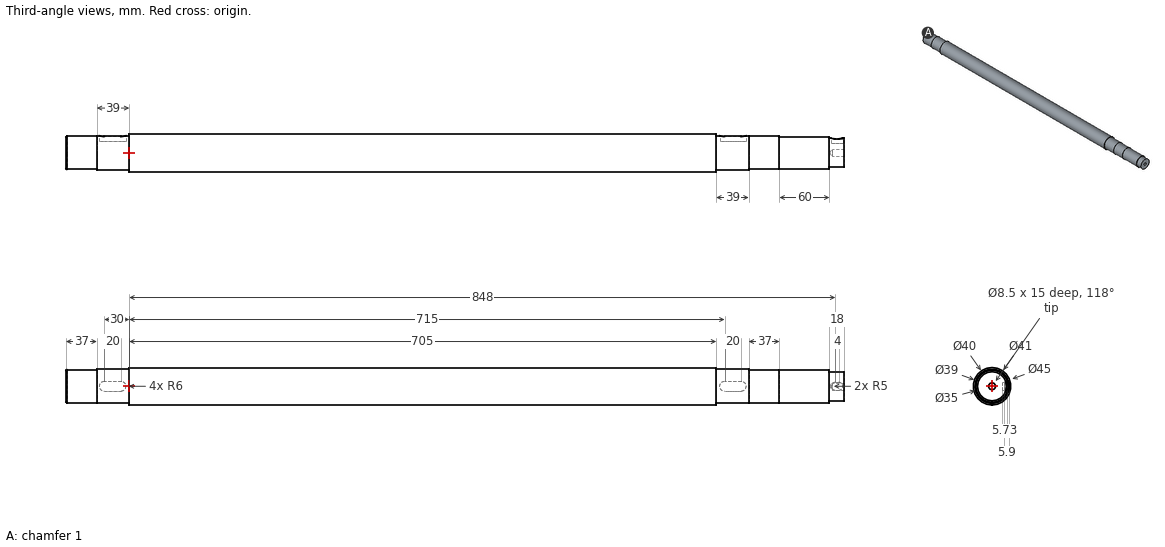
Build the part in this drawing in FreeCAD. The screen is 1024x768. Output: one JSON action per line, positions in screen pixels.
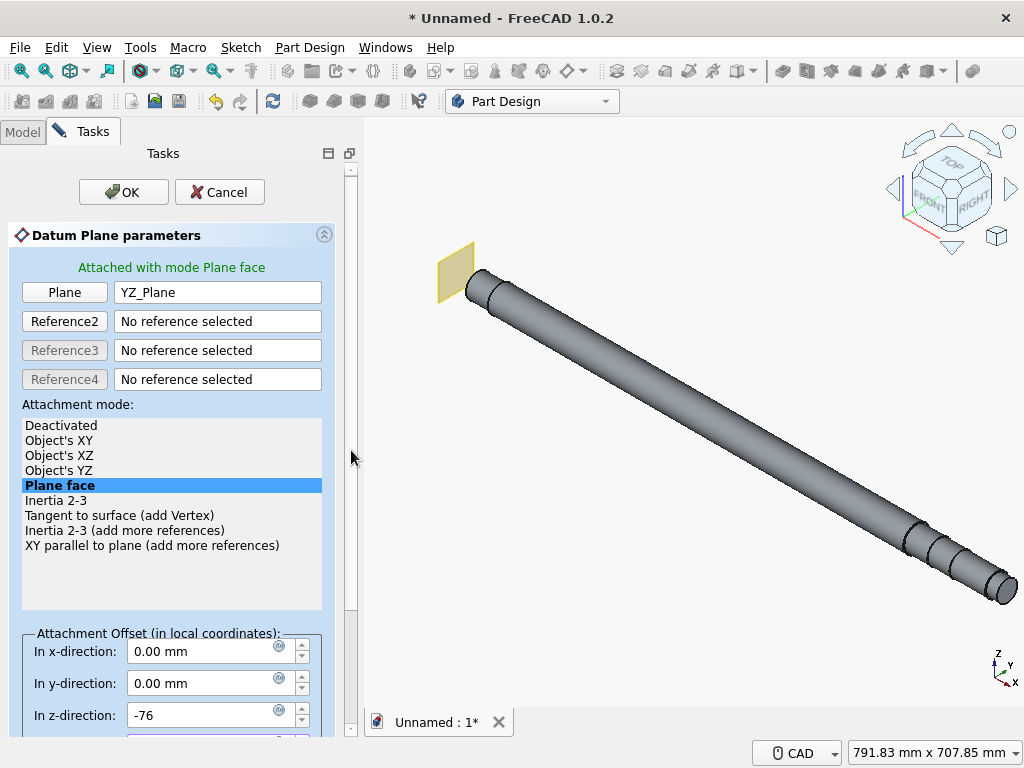
{"action": "left_click", "coordinate": [124, 192]}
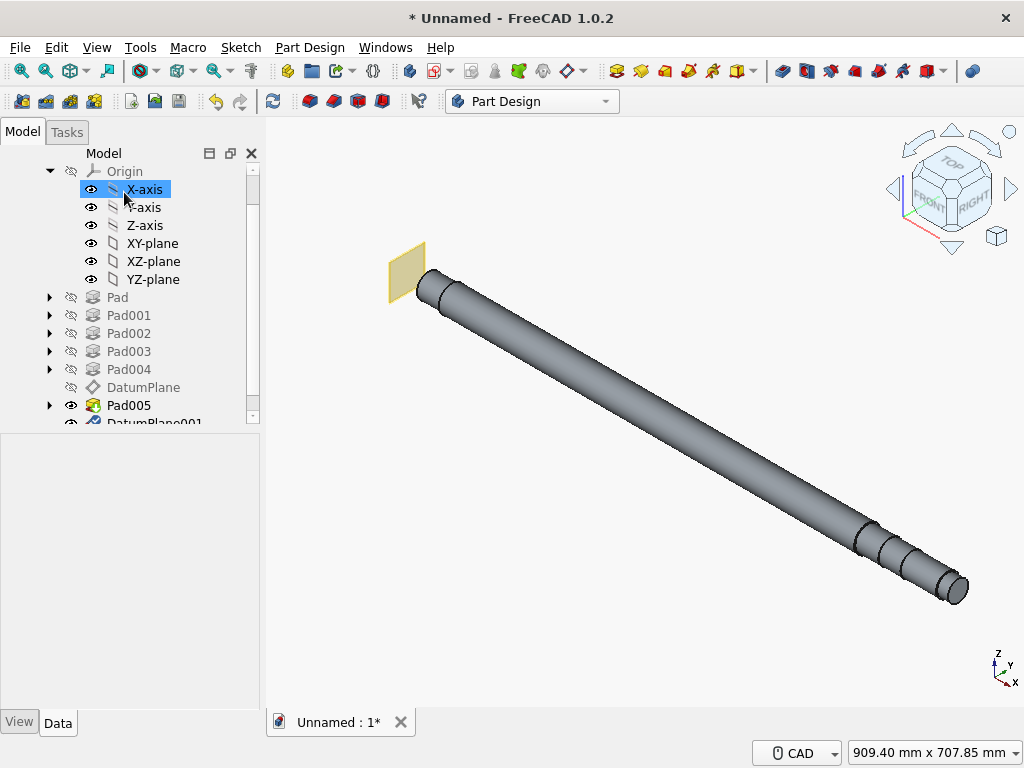
{"action": "left_click", "coordinate": [116, 423]}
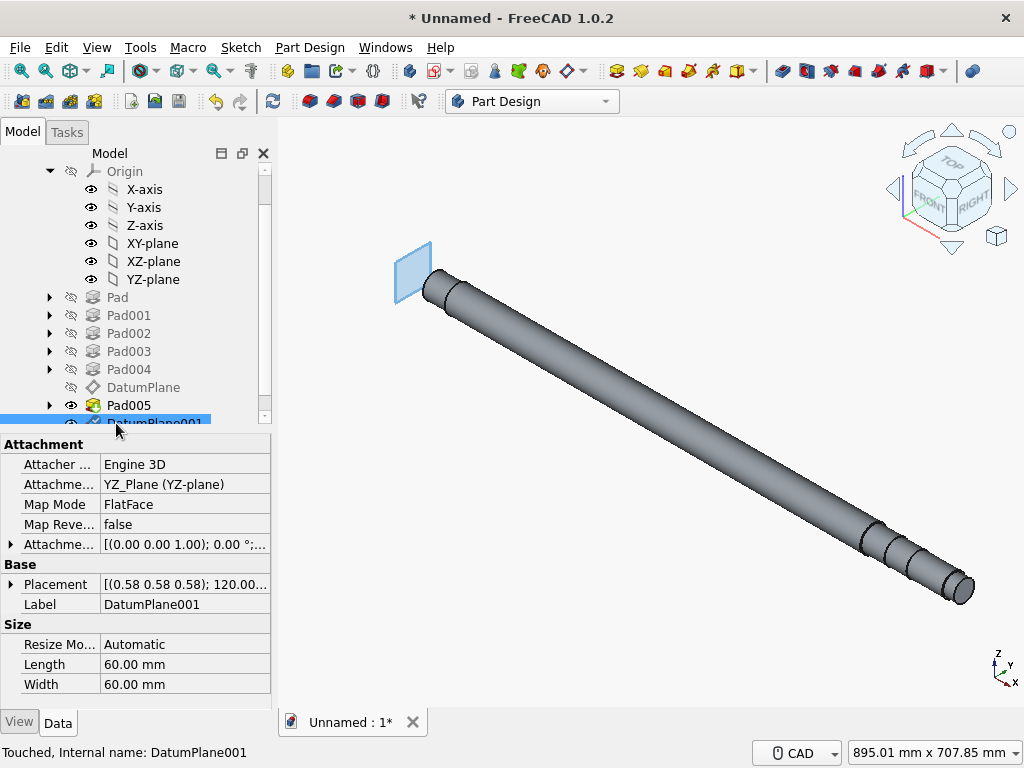
{"action": "left_click", "coordinate": [434, 72]}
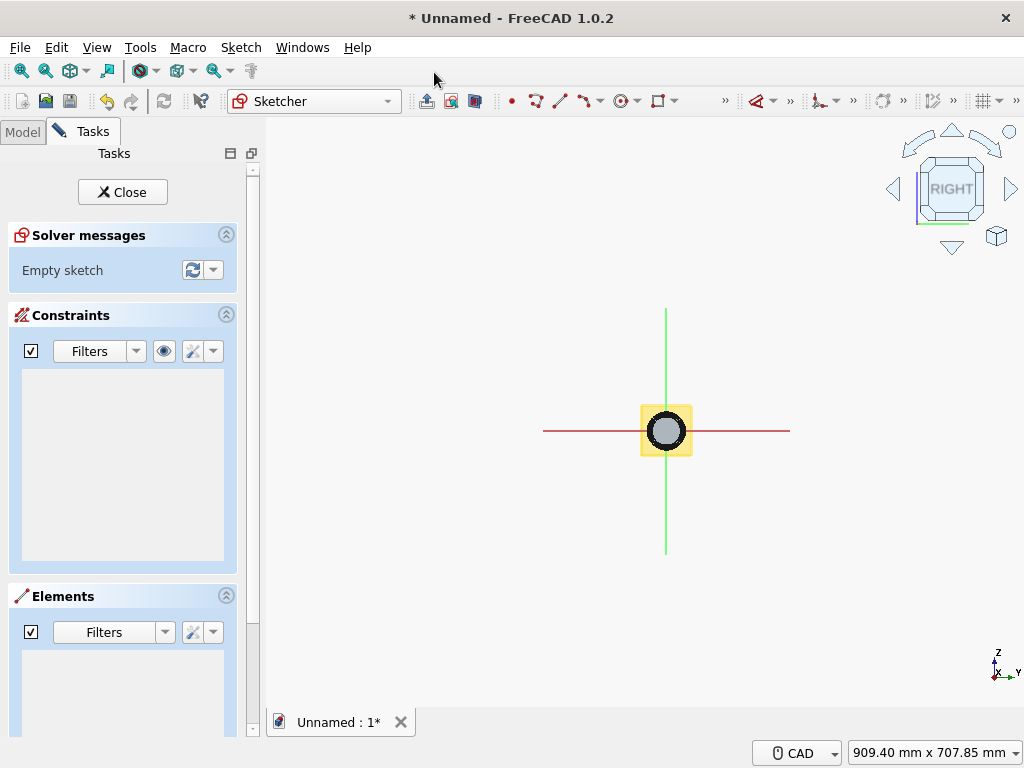
{"action": "left_click", "coordinate": [476, 102]}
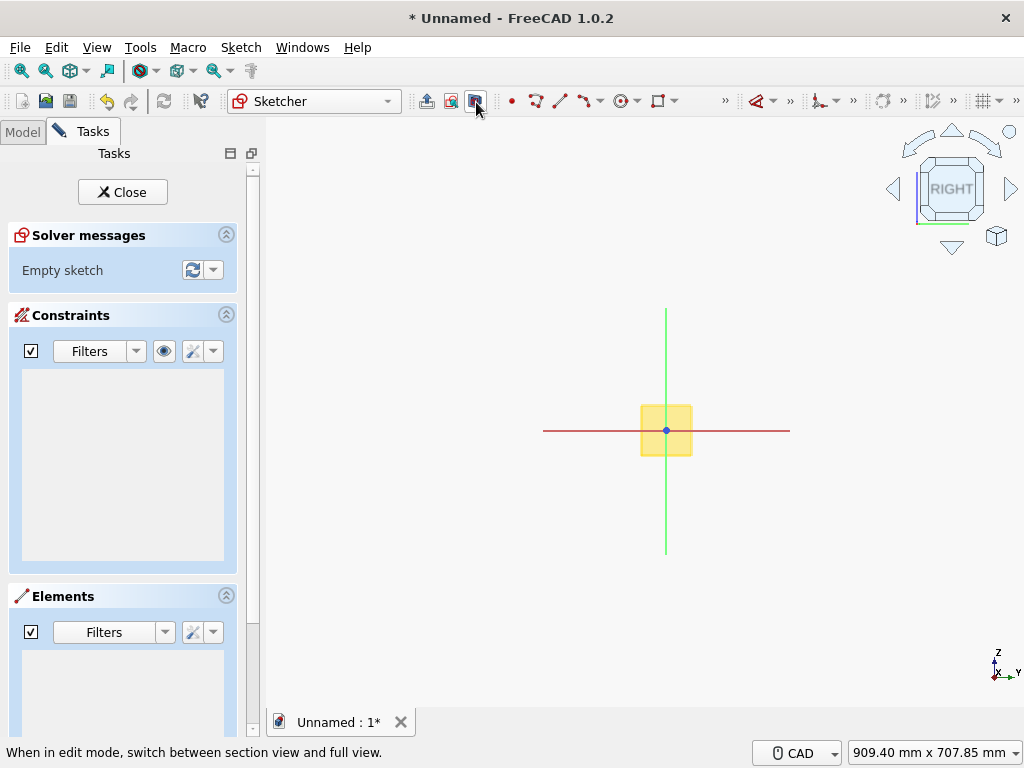
{"action": "scroll", "coordinate": [675, 433], "scroll_direction": "up", "scroll_amount": 12}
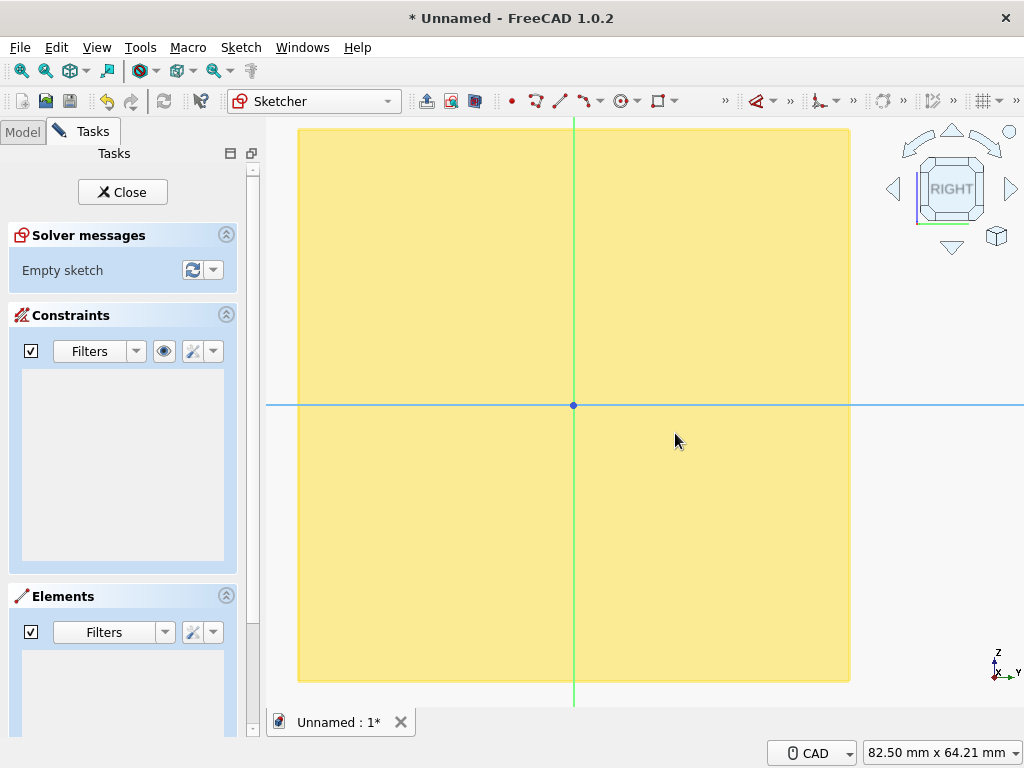
{"action": "left_click", "coordinate": [622, 102]}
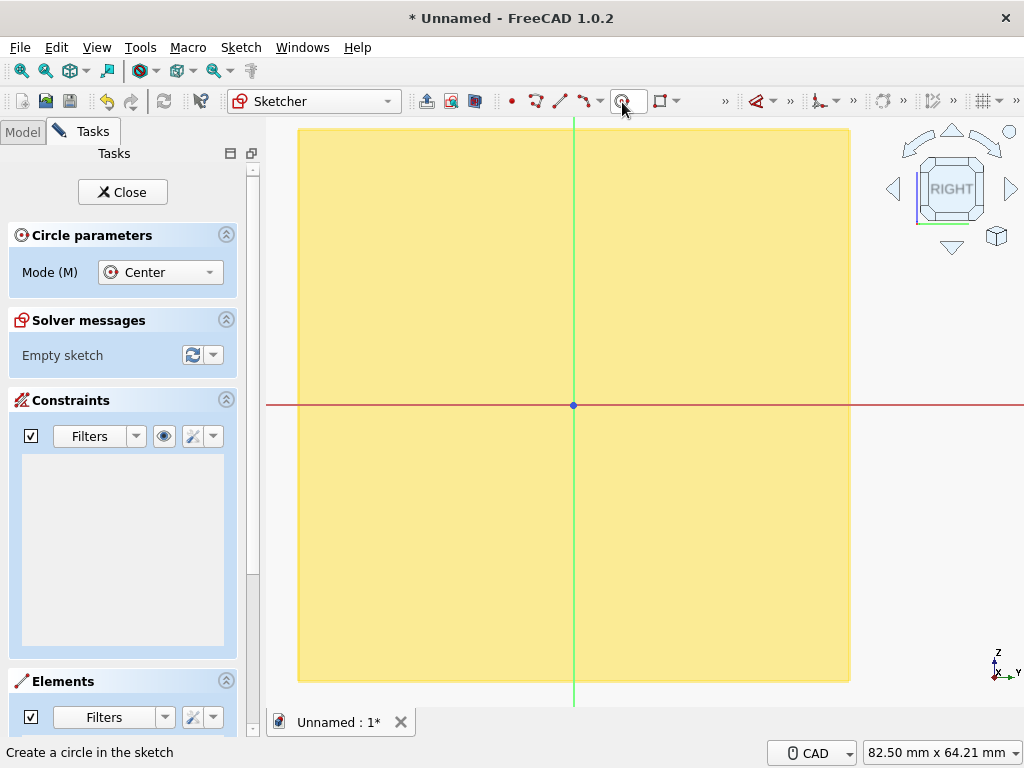
{"action": "left_click", "coordinate": [574, 405]}
{"action": "mouse_move", "coordinate": [704, 276]}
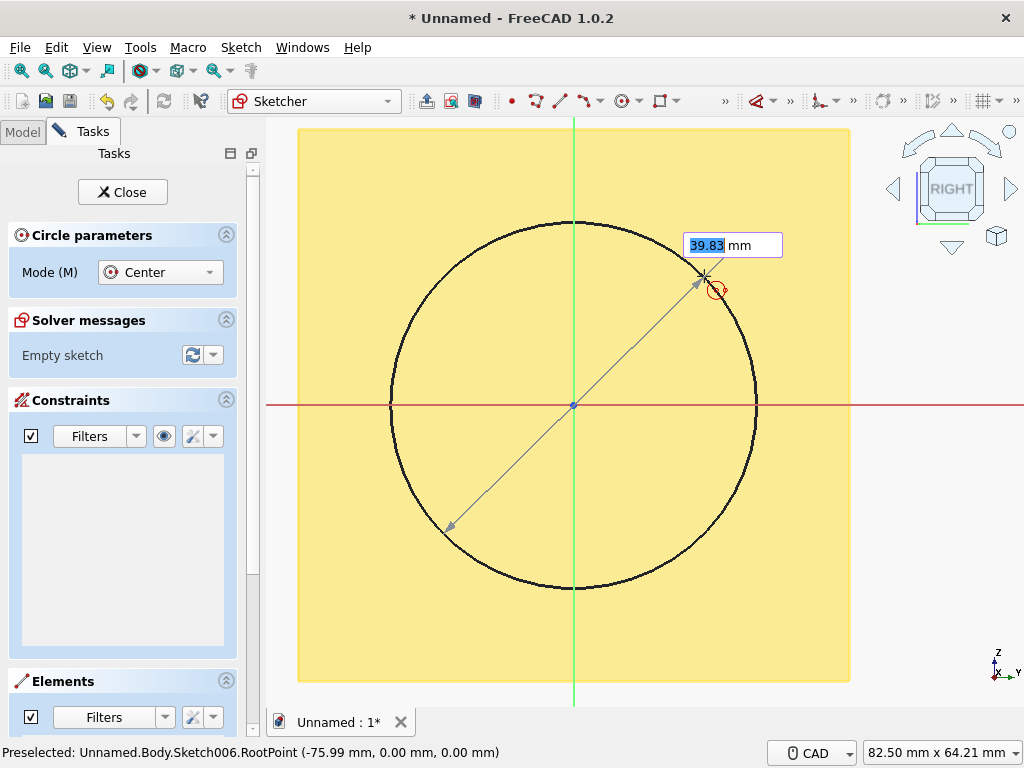
{"action": "type", "text": "40"}
{"action": "key", "text": "Return"}
{"action": "key", "text": "Escape"}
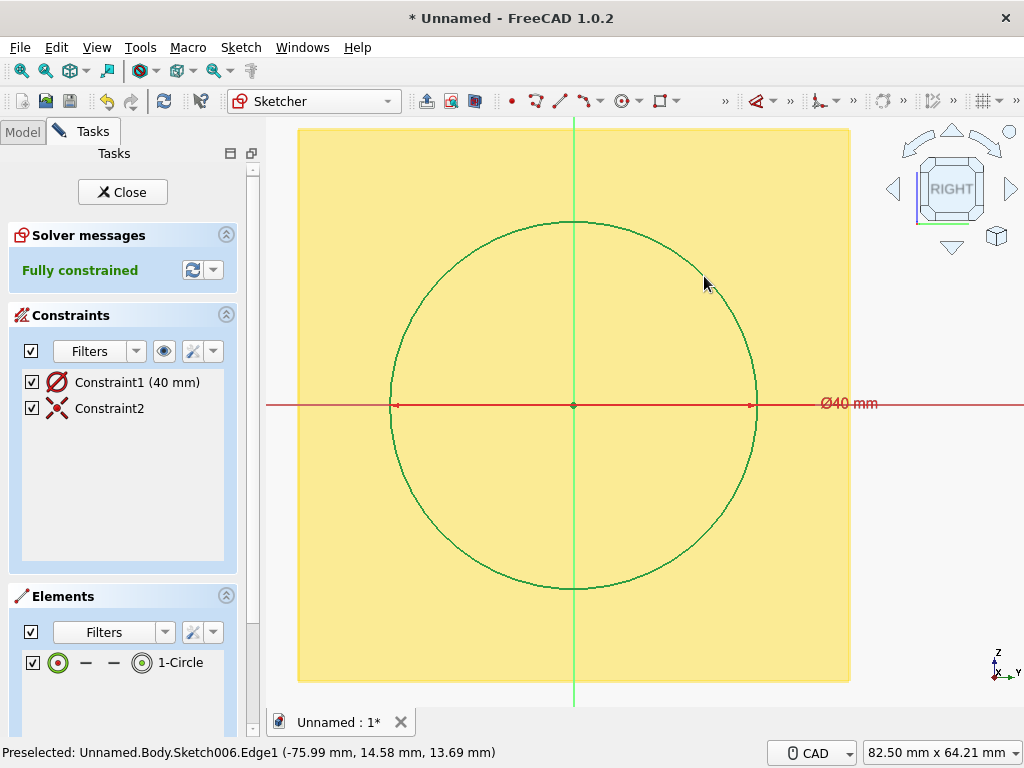
{"action": "left_click", "coordinate": [123, 192]}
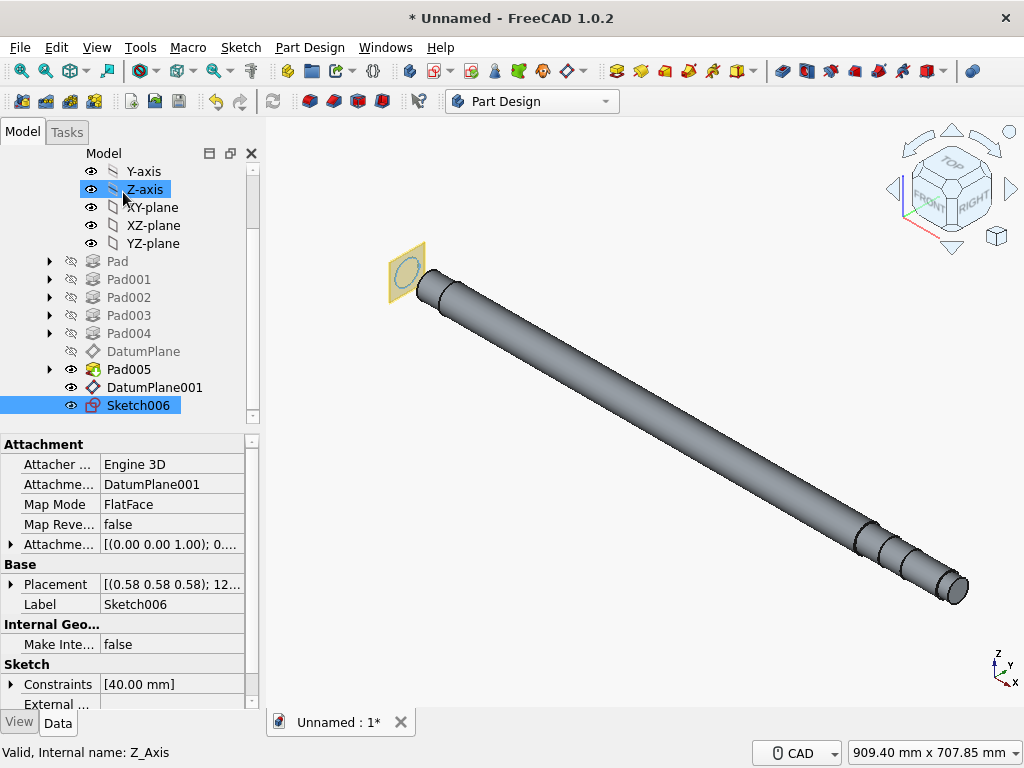
{"action": "left_click", "coordinate": [618, 72]}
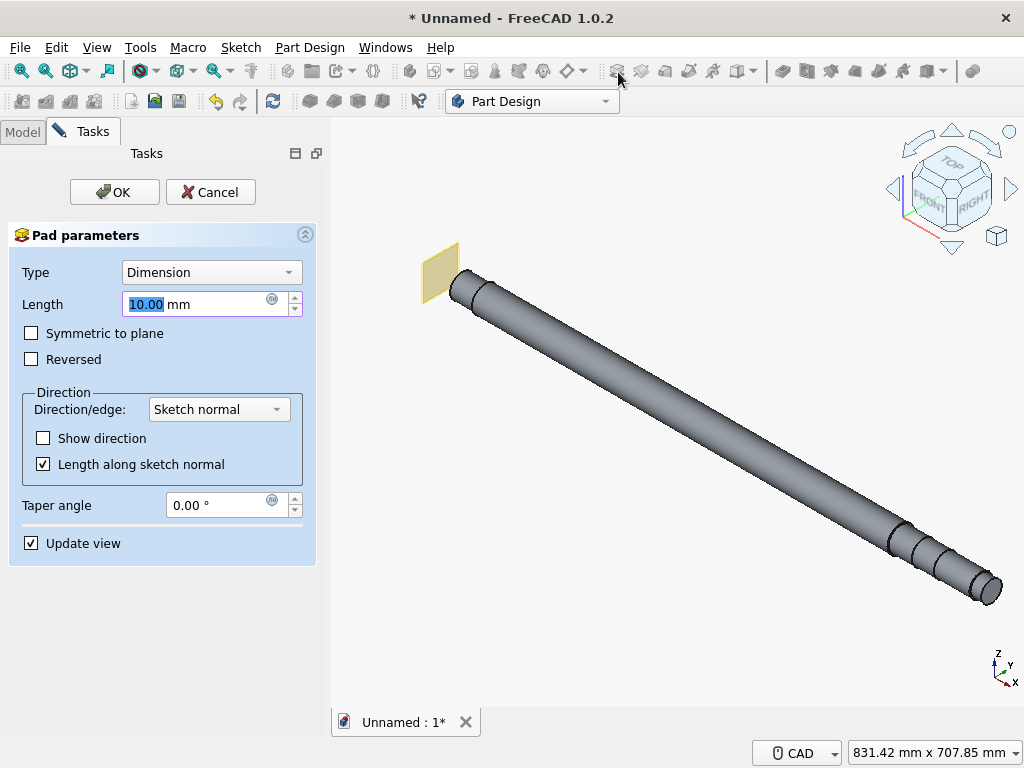
{"action": "type", "text": "37"}
{"action": "key", "text": "Tab"}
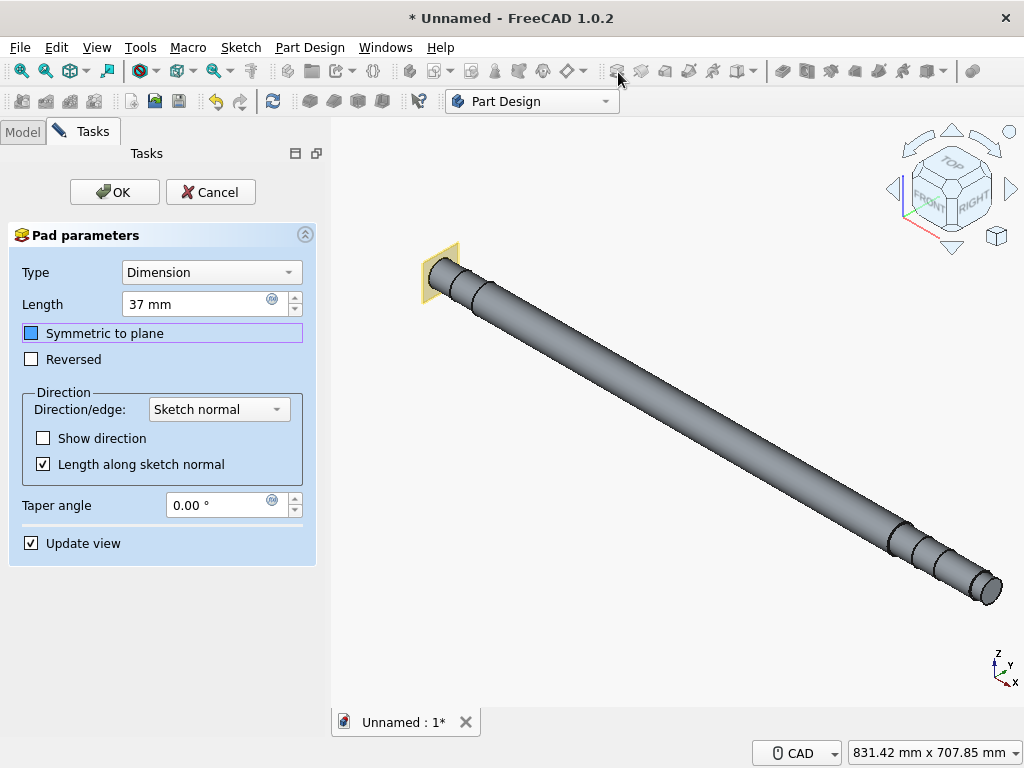
{"action": "left_click", "coordinate": [115, 192]}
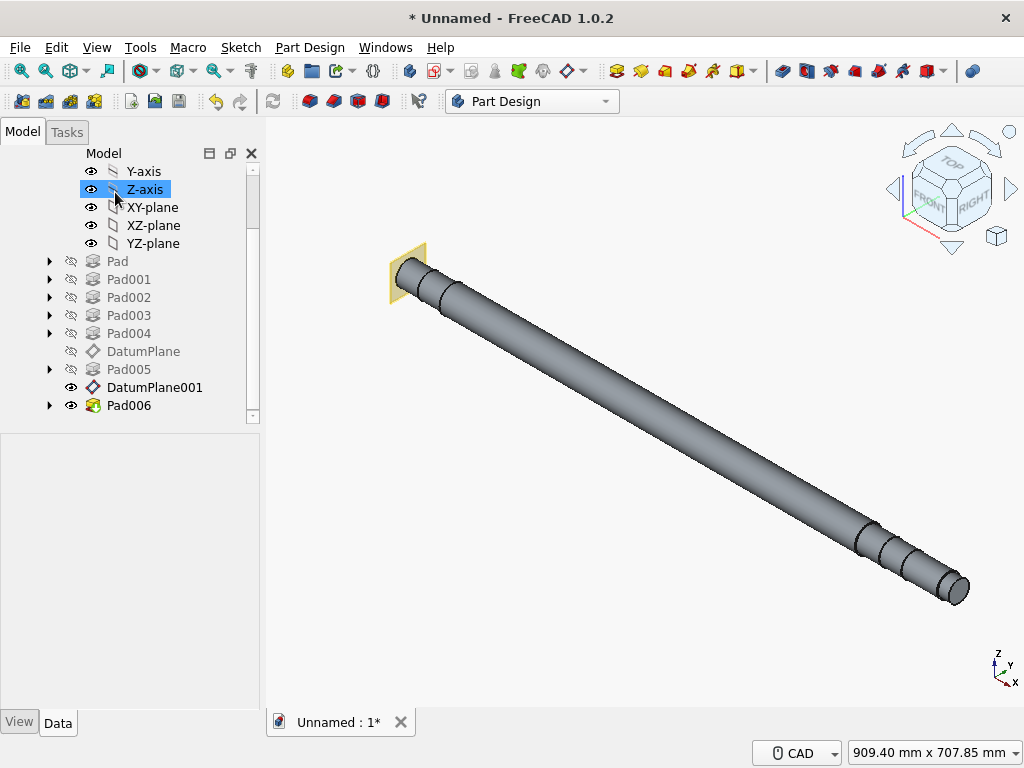
{"action": "left_click", "coordinate": [116, 387]}
{"action": "key", "text": "space"}